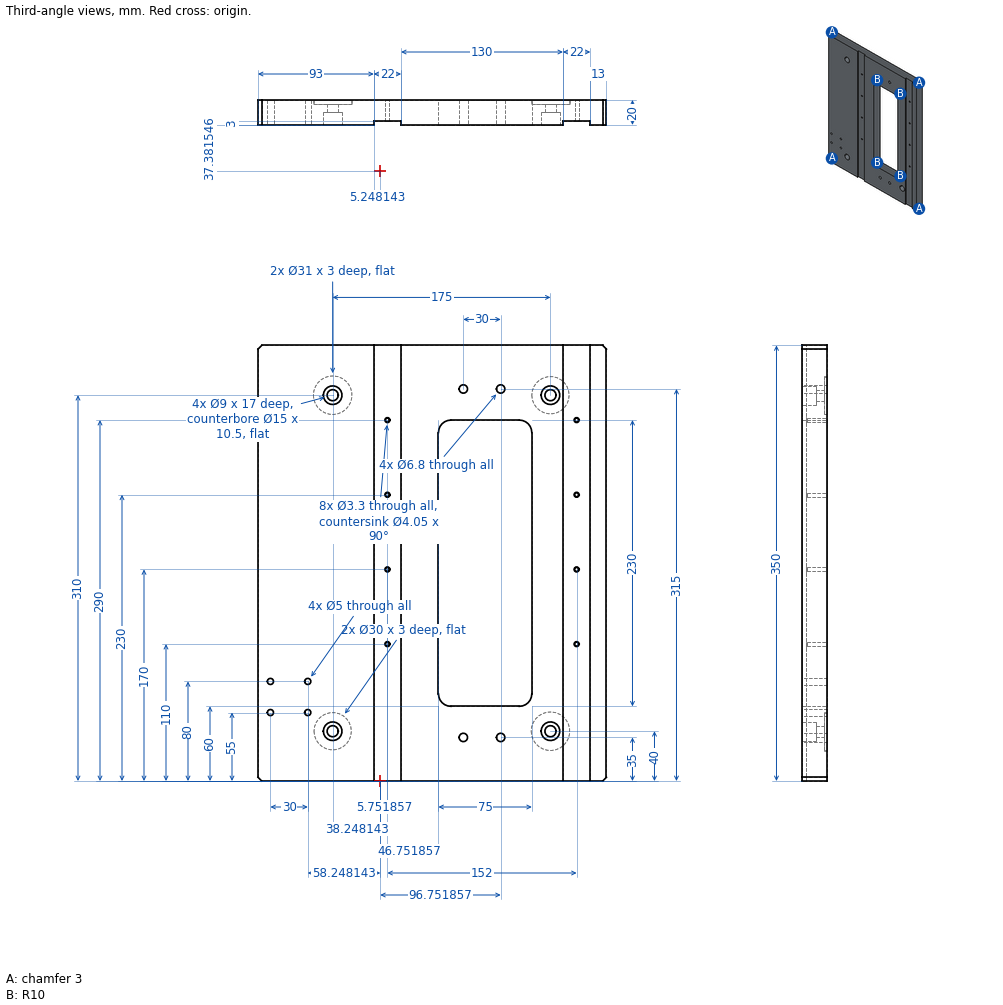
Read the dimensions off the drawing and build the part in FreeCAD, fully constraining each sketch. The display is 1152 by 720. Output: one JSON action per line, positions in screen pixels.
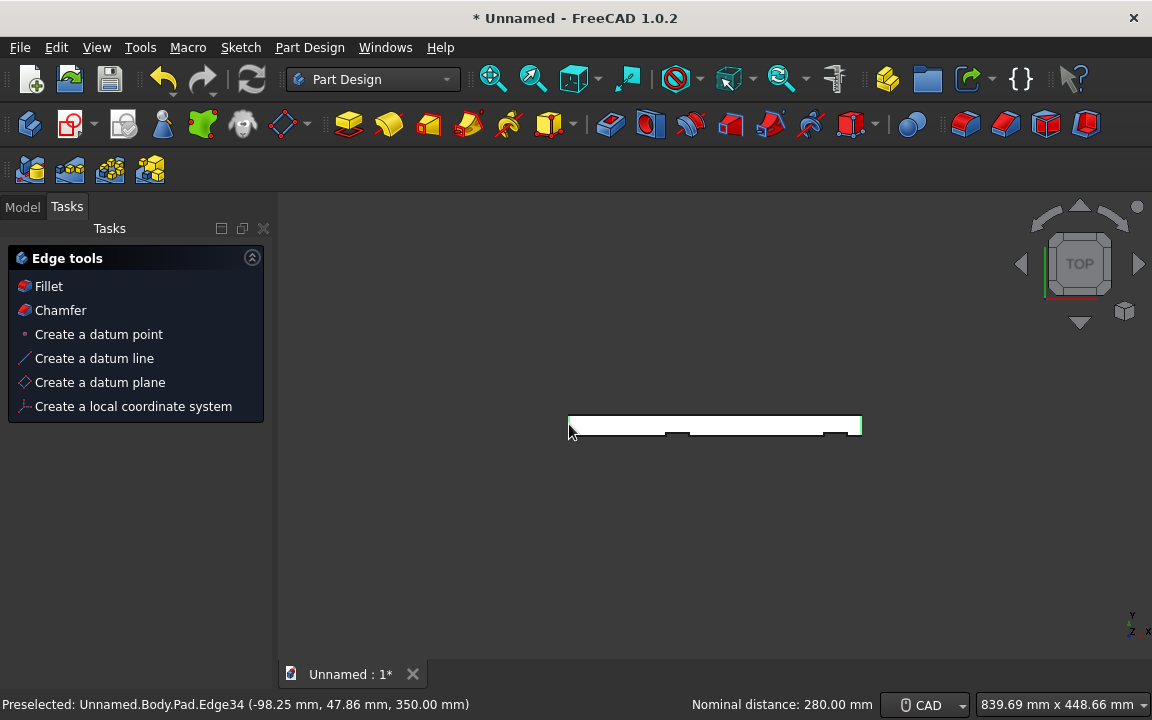
{"action": "scroll", "coordinate": [861, 424], "scroll_direction": "up", "scroll_amount": 4}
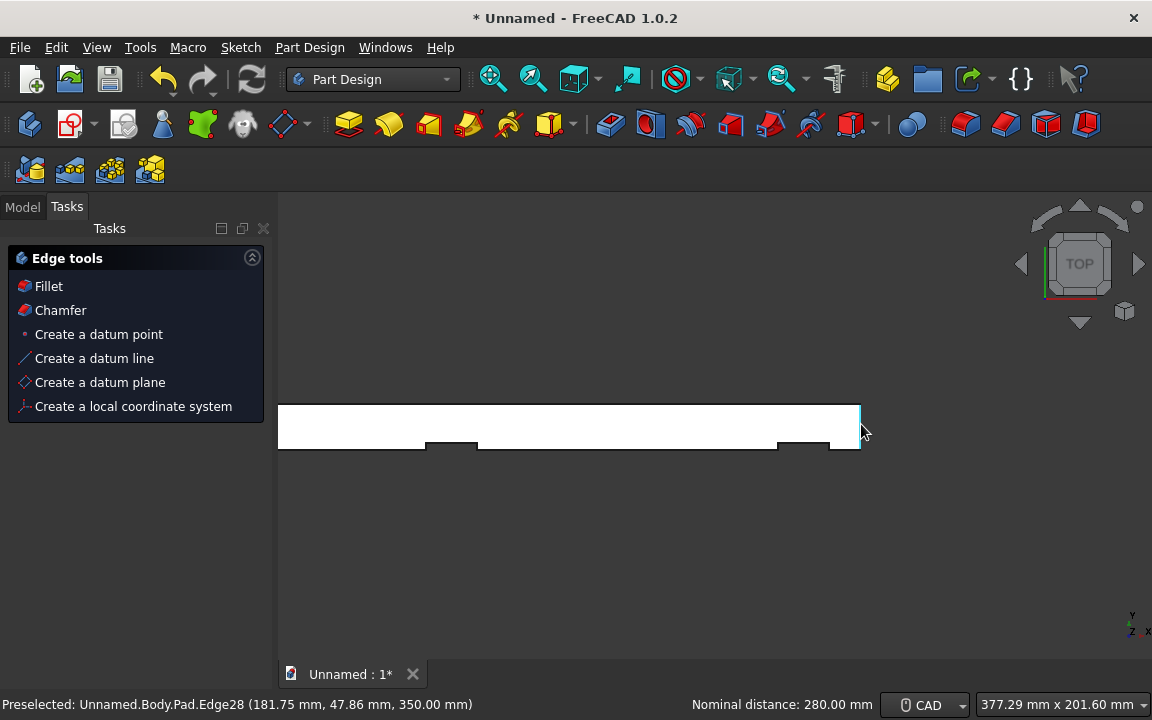
{"action": "left_click", "coordinate": [494, 80]}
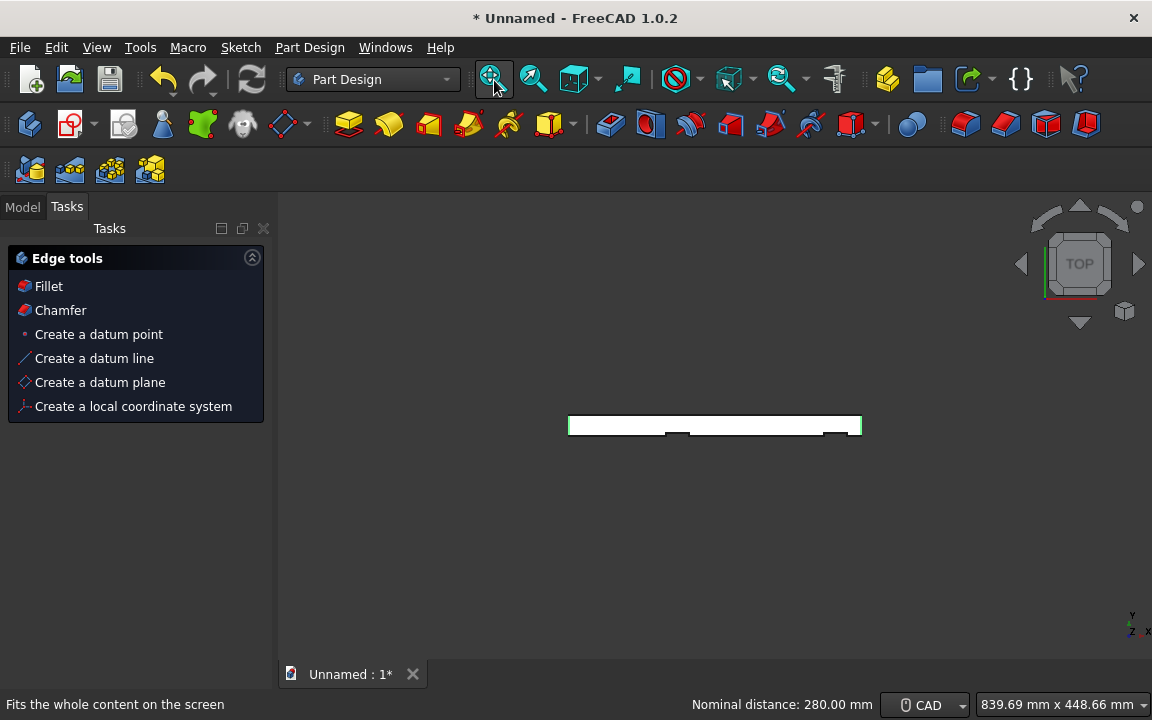
{"action": "key", "text": "1"}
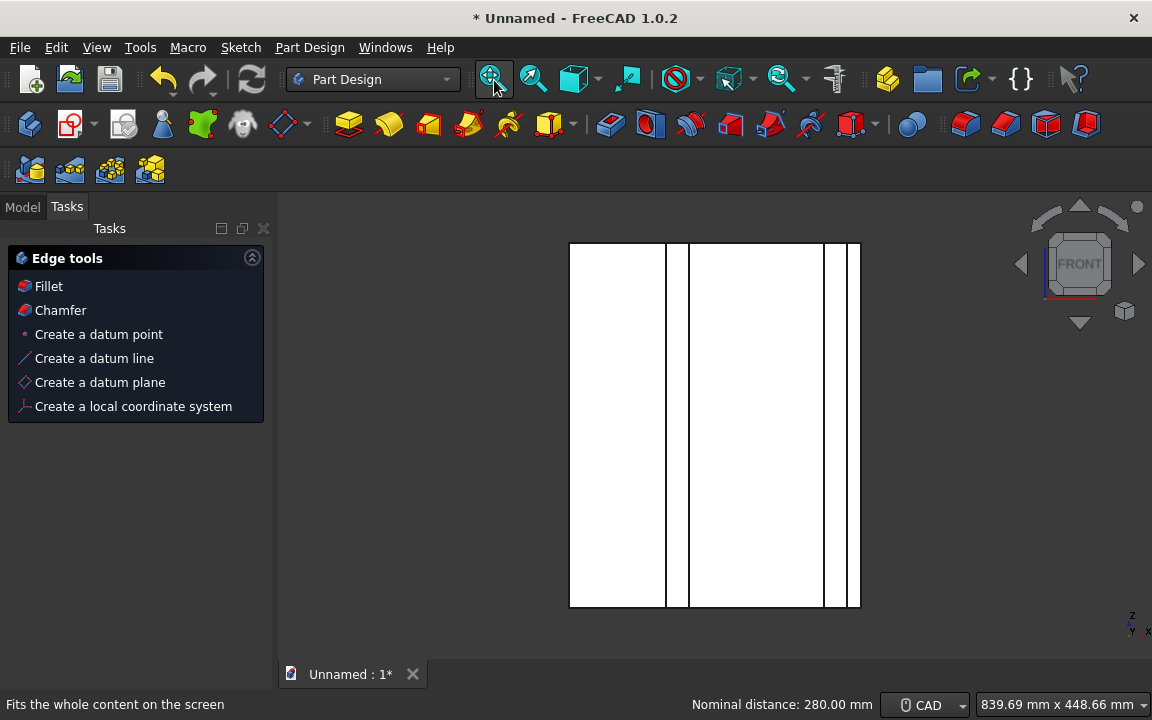
{"action": "scroll", "coordinate": [861, 607], "scroll_direction": "up", "scroll_amount": 4}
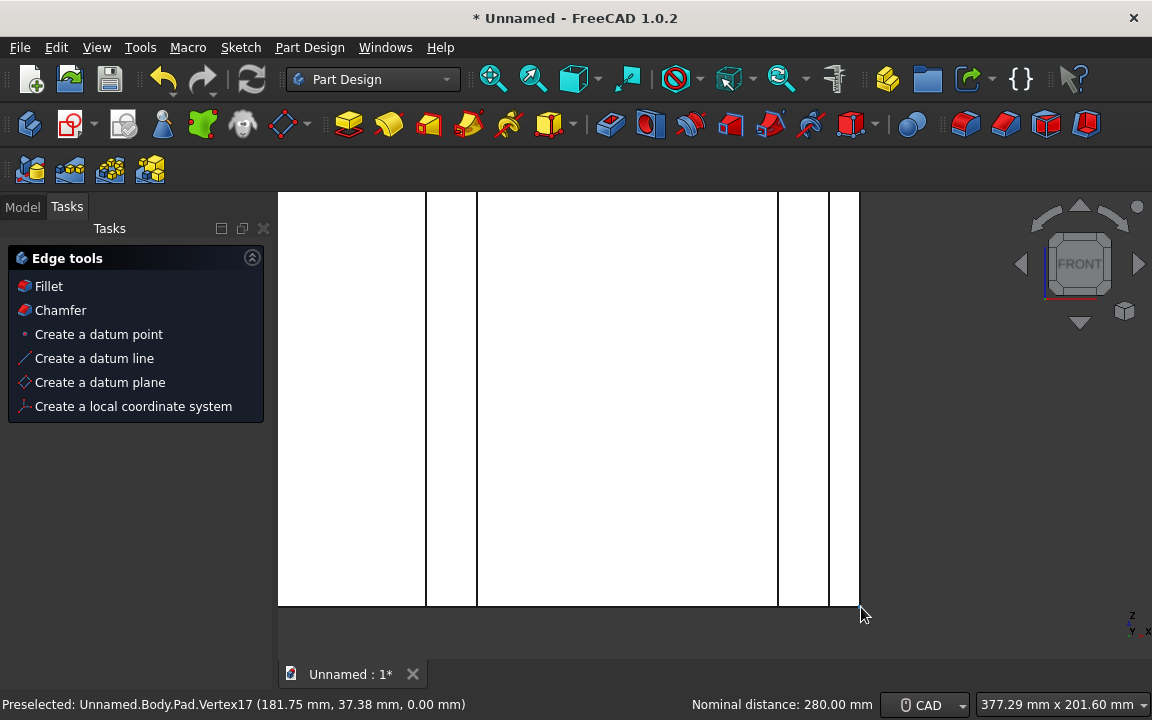
{"action": "left_click", "coordinate": [494, 80]}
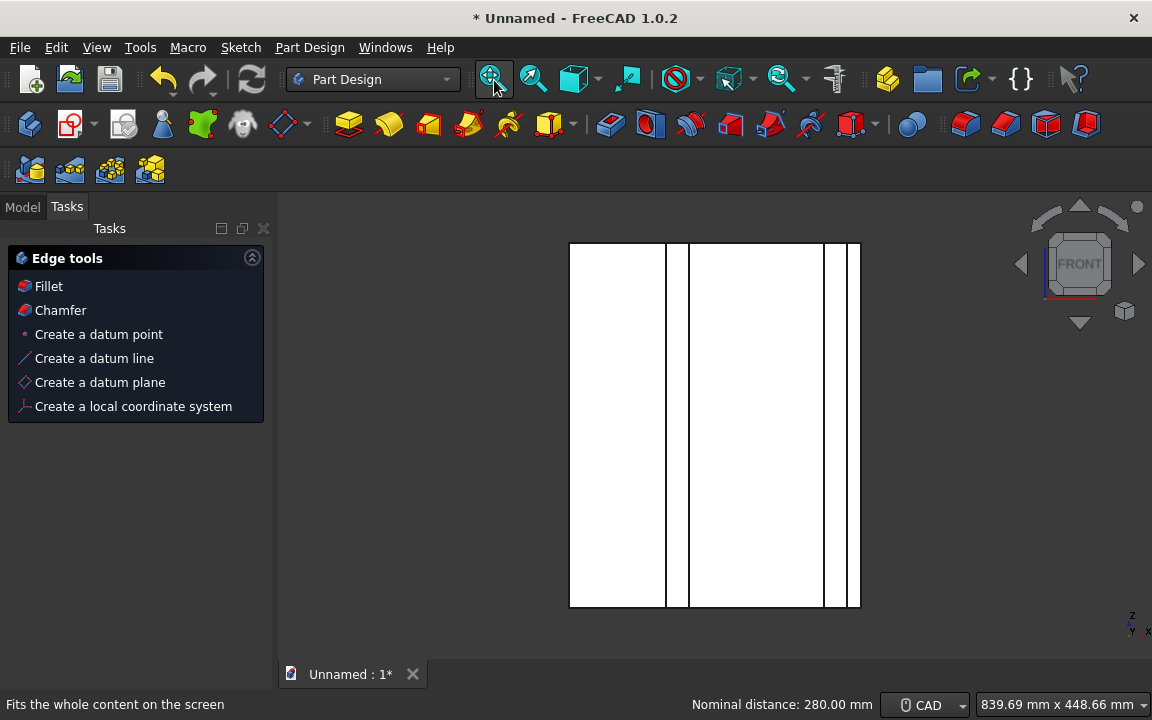
{"action": "key", "text": "3"}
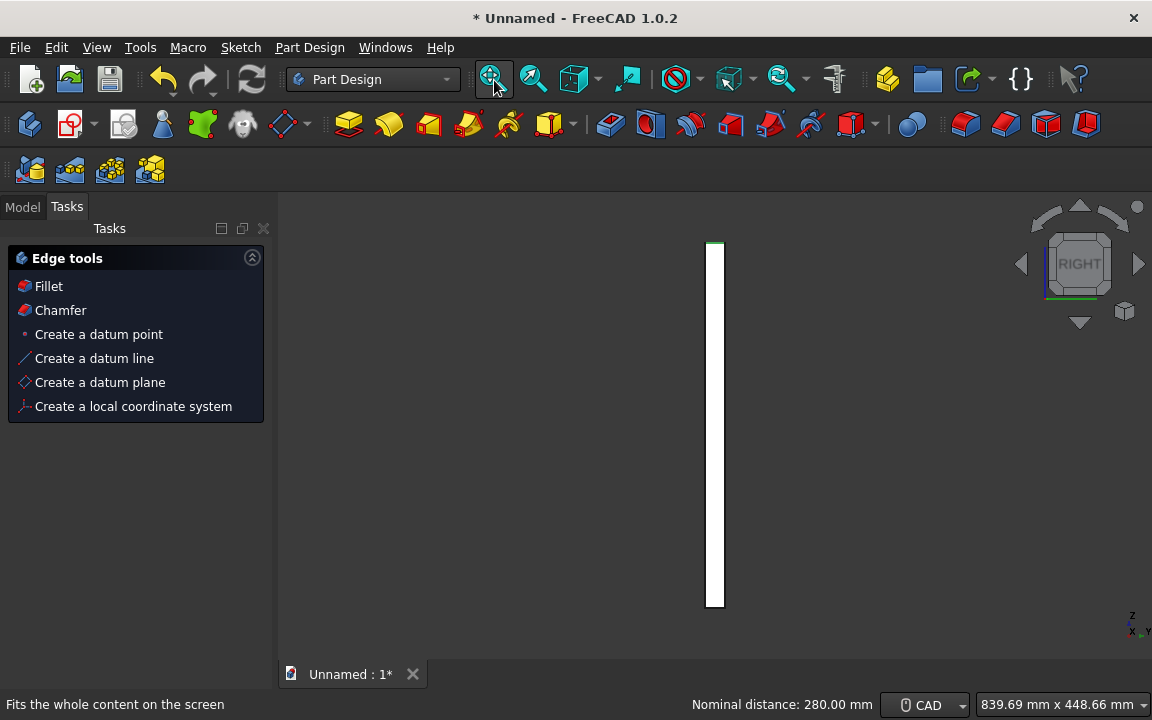
{"action": "left_click", "coordinate": [715, 607], "text": "ctrl"}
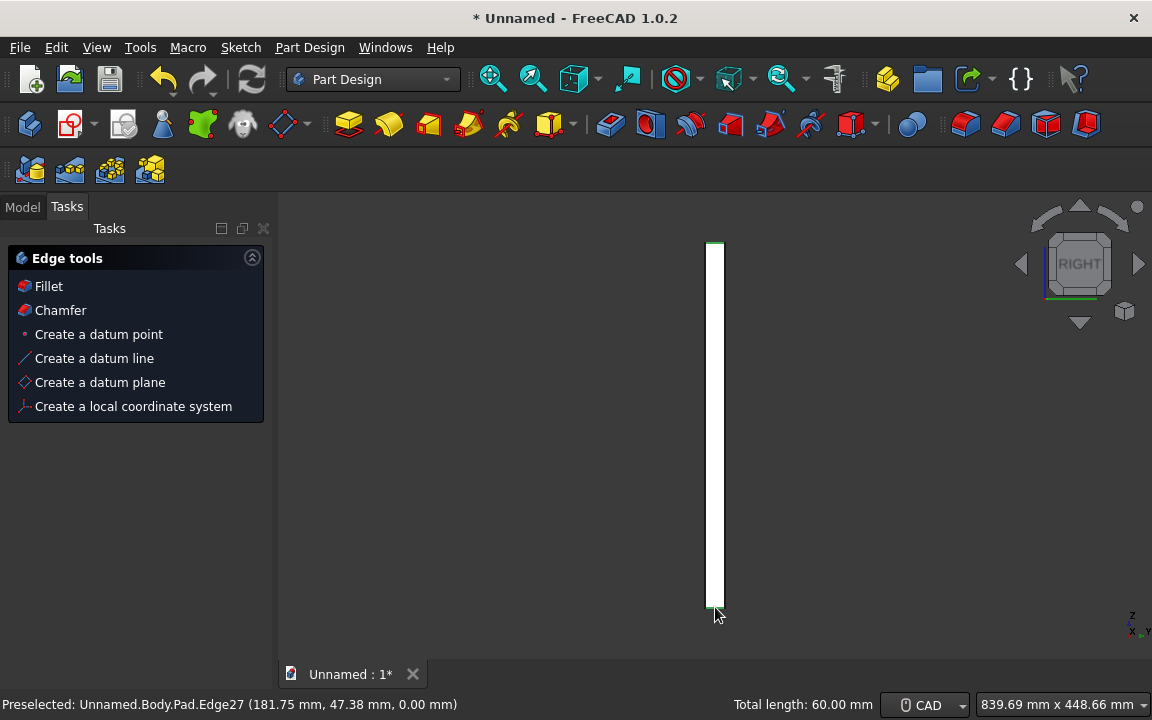
{"action": "scroll", "coordinate": [715, 607], "scroll_direction": "up", "scroll_amount": 4}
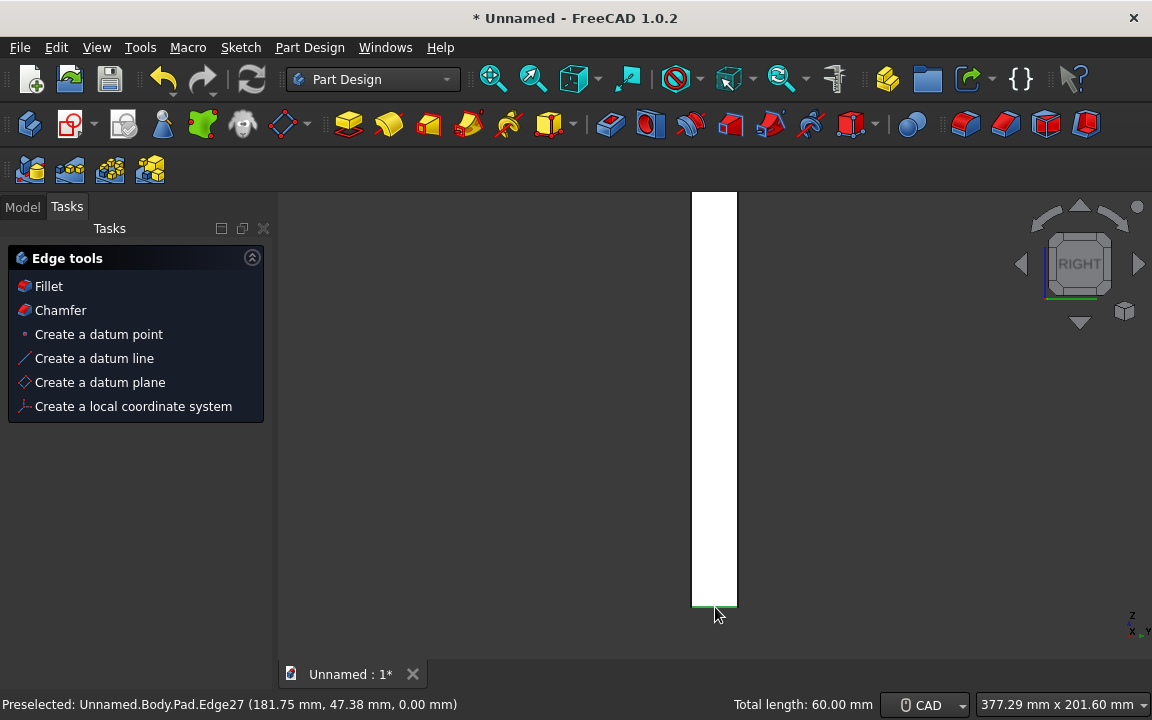
{"action": "left_click", "coordinate": [494, 80]}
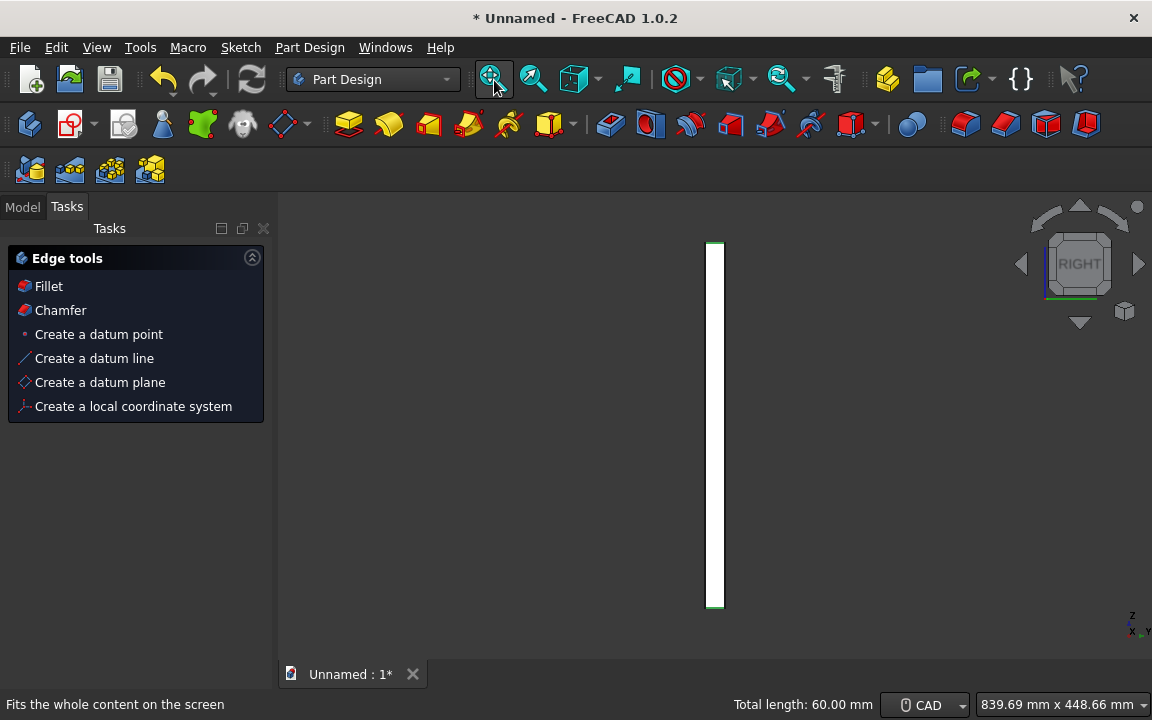
{"action": "key", "text": "5"}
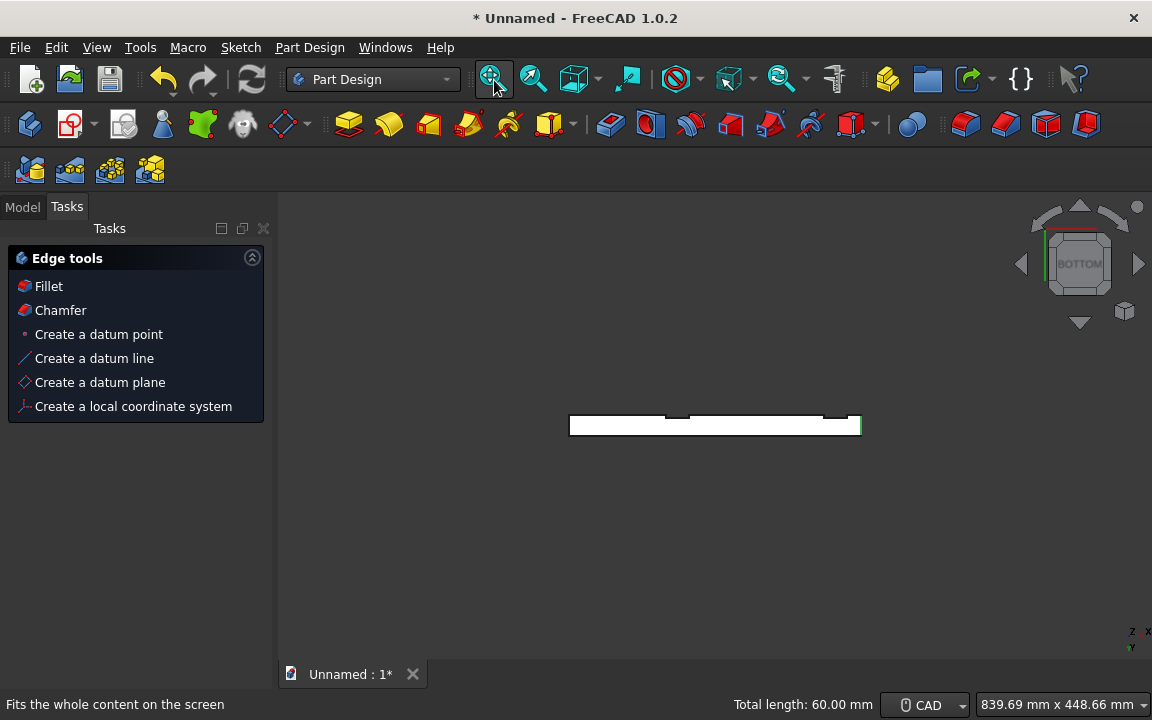
{"action": "left_click", "coordinate": [494, 80]}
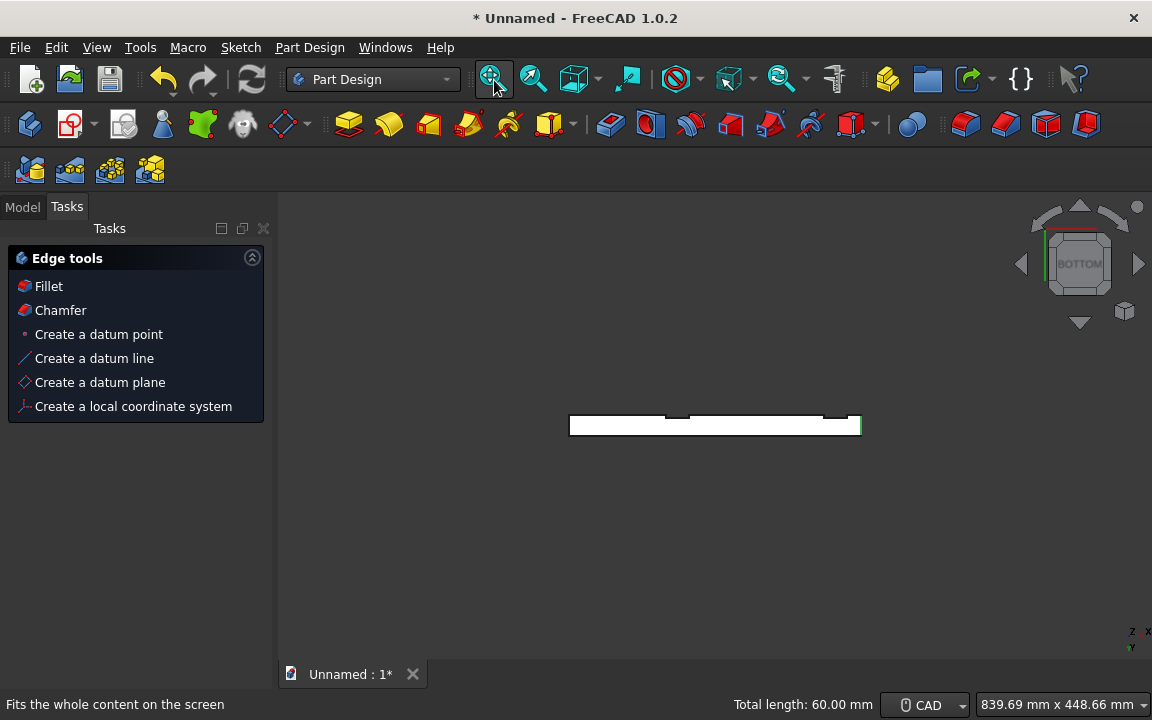
{"action": "left_click", "coordinate": [569, 424], "text": "ctrl"}